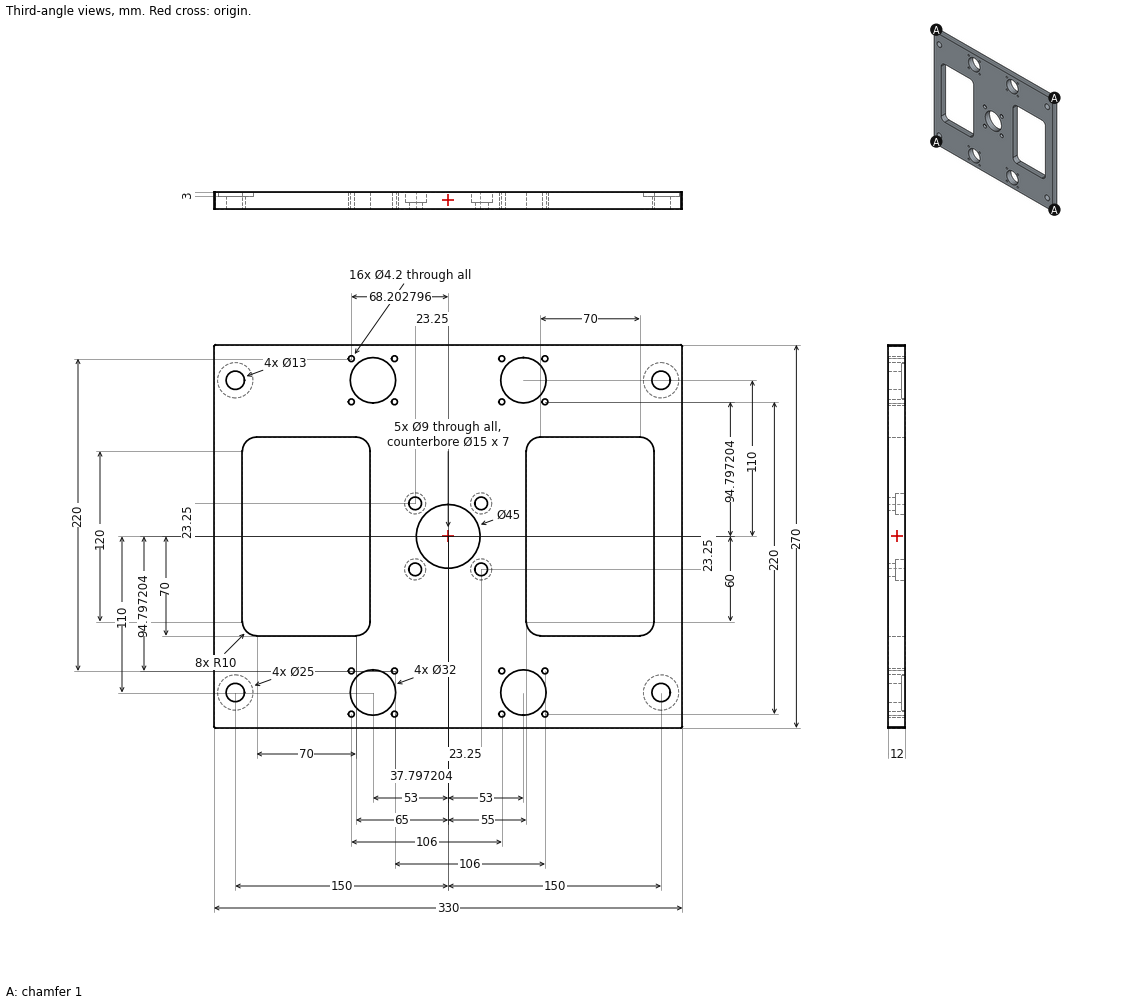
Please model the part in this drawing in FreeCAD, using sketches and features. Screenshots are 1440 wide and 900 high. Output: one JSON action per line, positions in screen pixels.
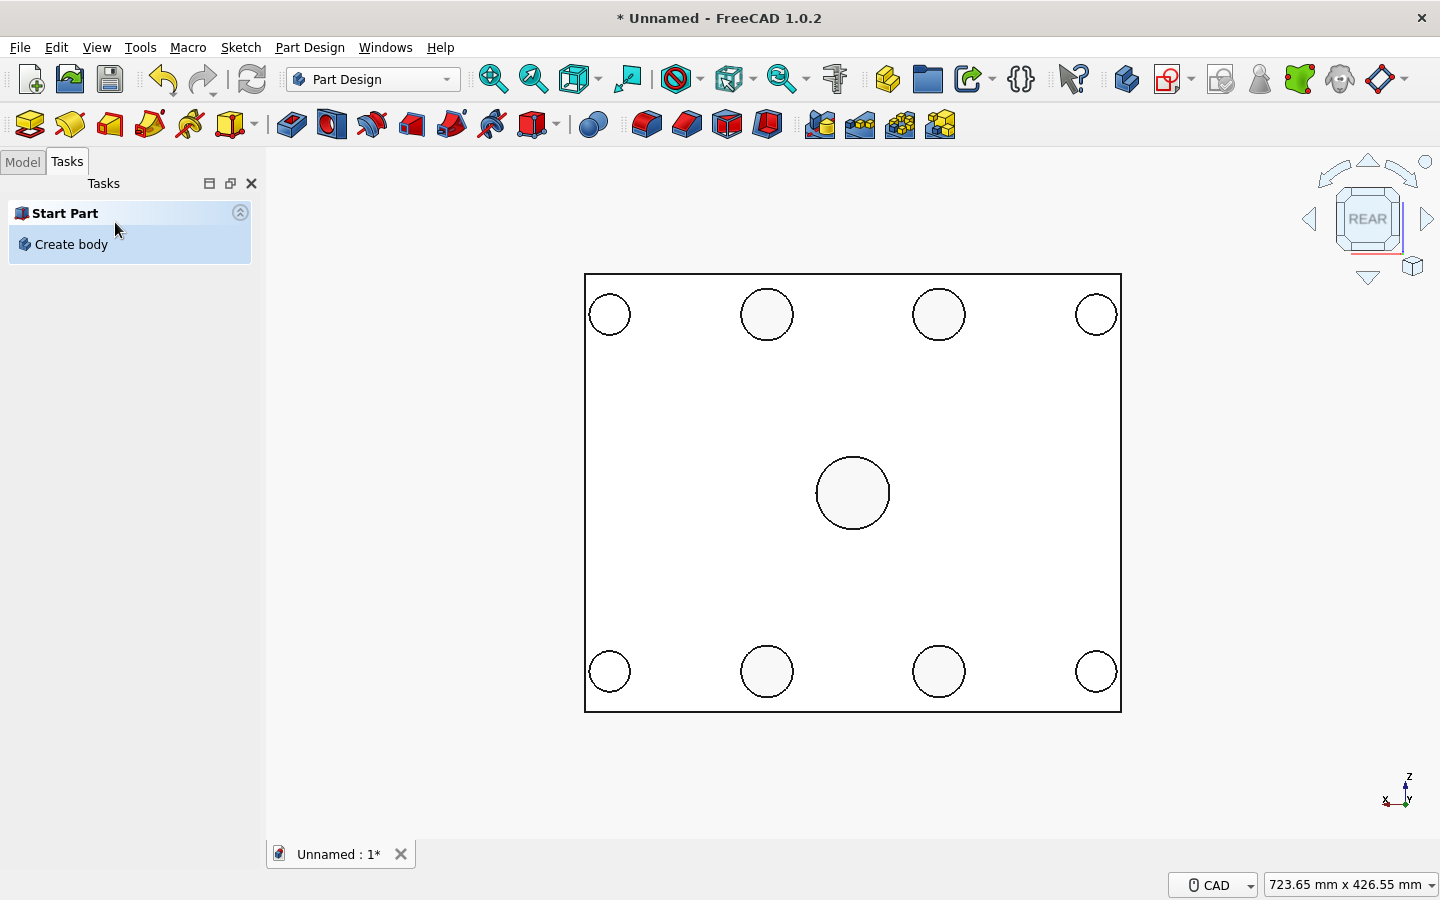
{"action": "key", "text": "0"}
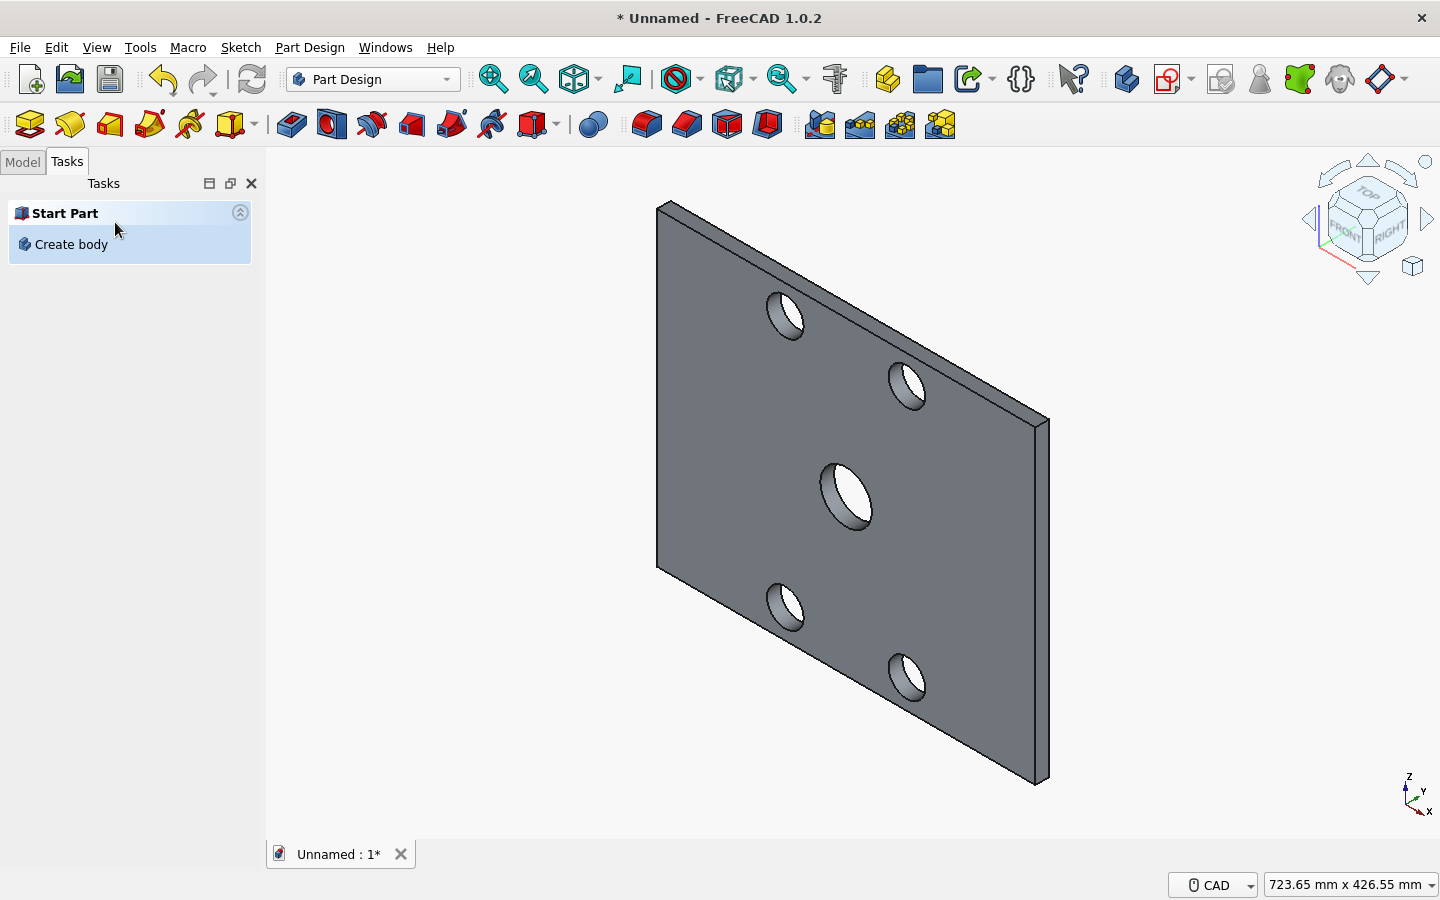
{"action": "left_click", "coordinate": [954, 558]}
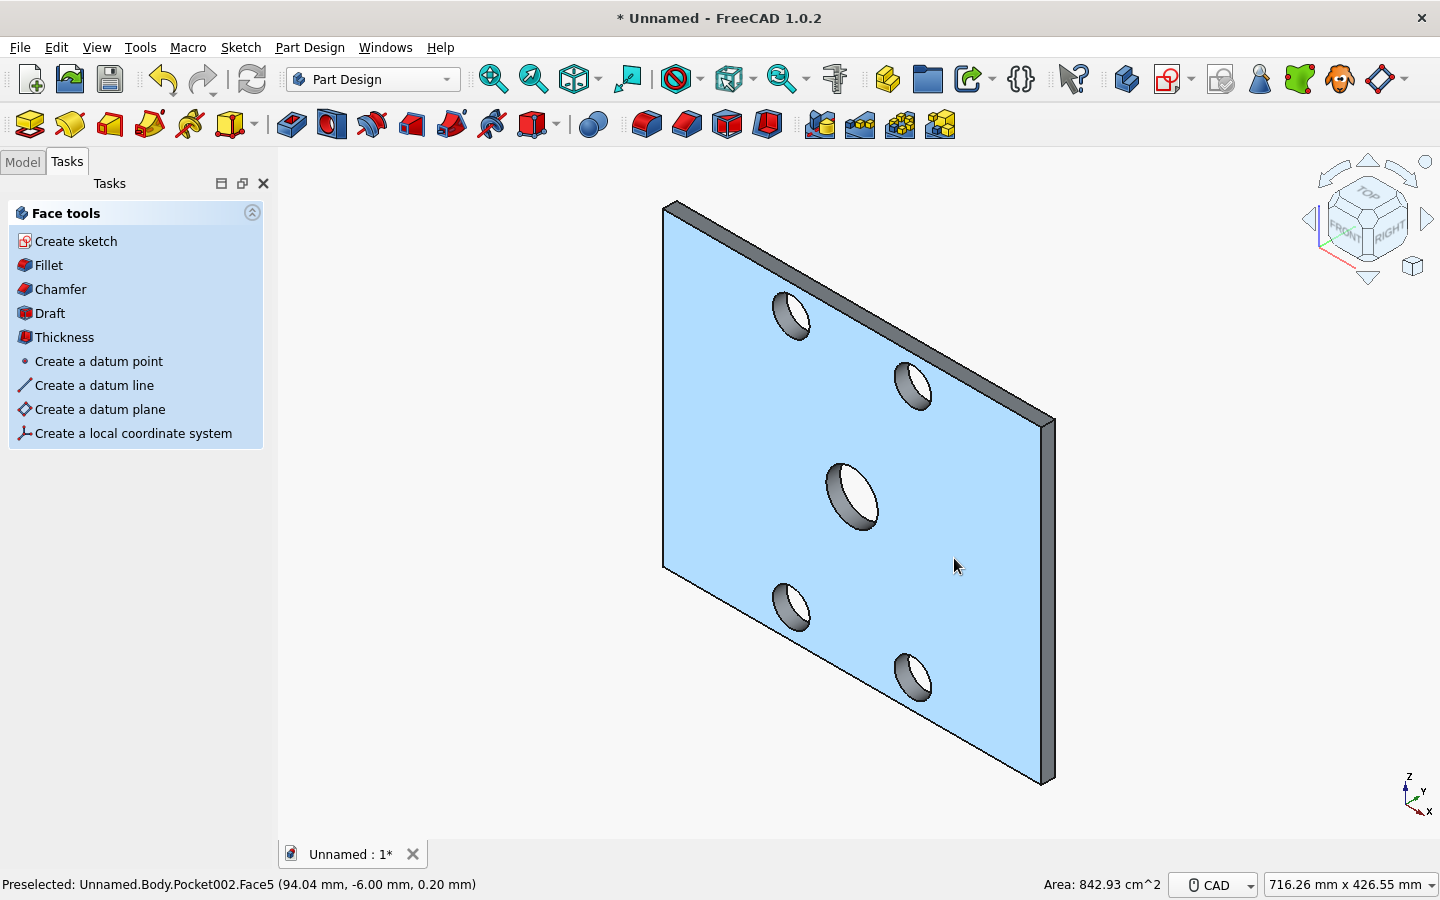
{"action": "left_click", "coordinate": [1168, 80]}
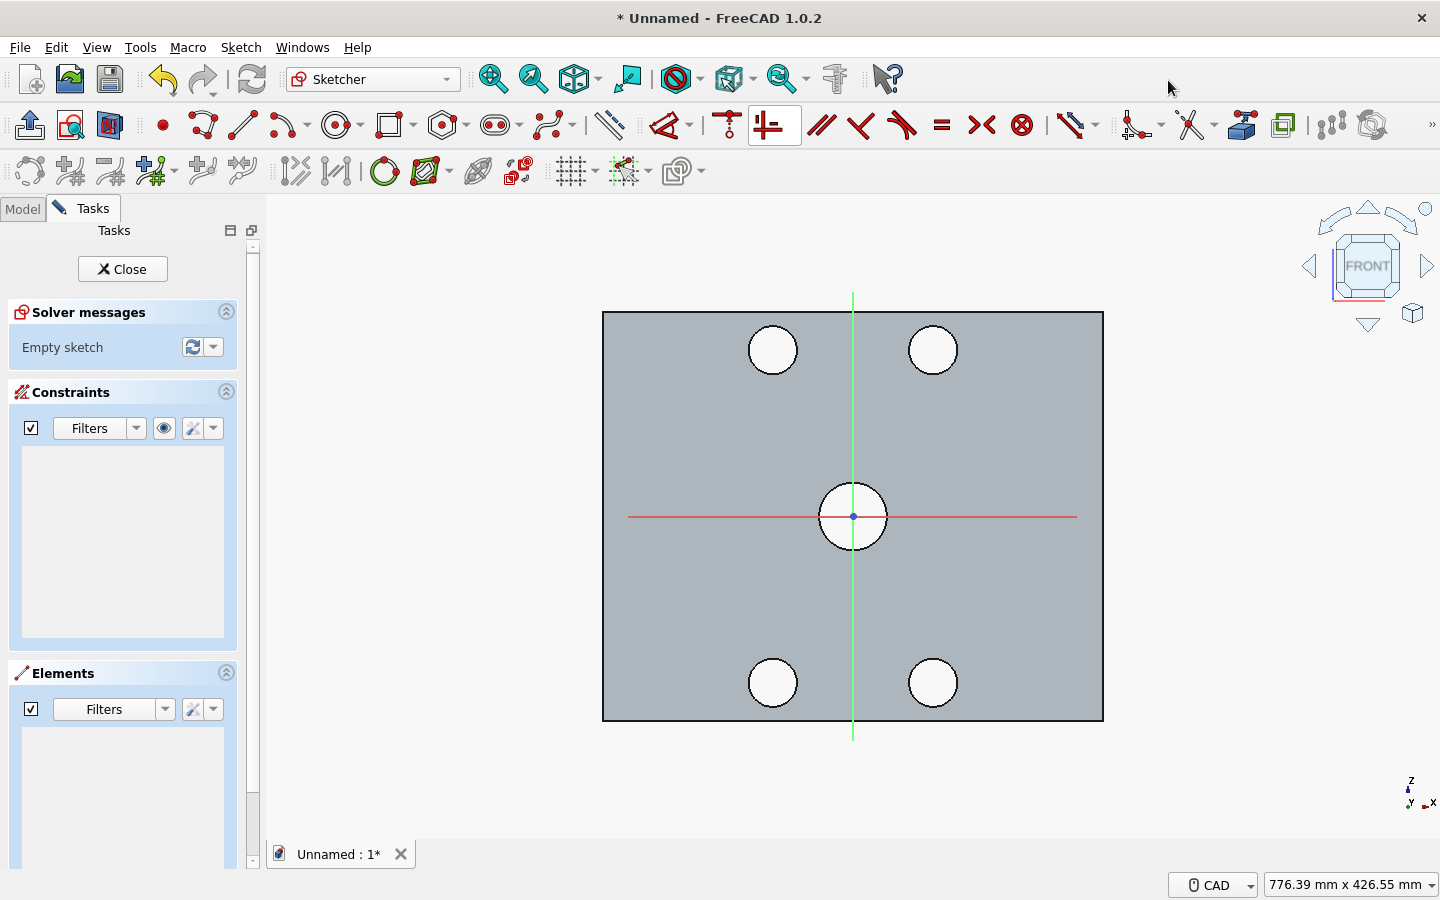
{"action": "left_click", "coordinate": [336, 126]}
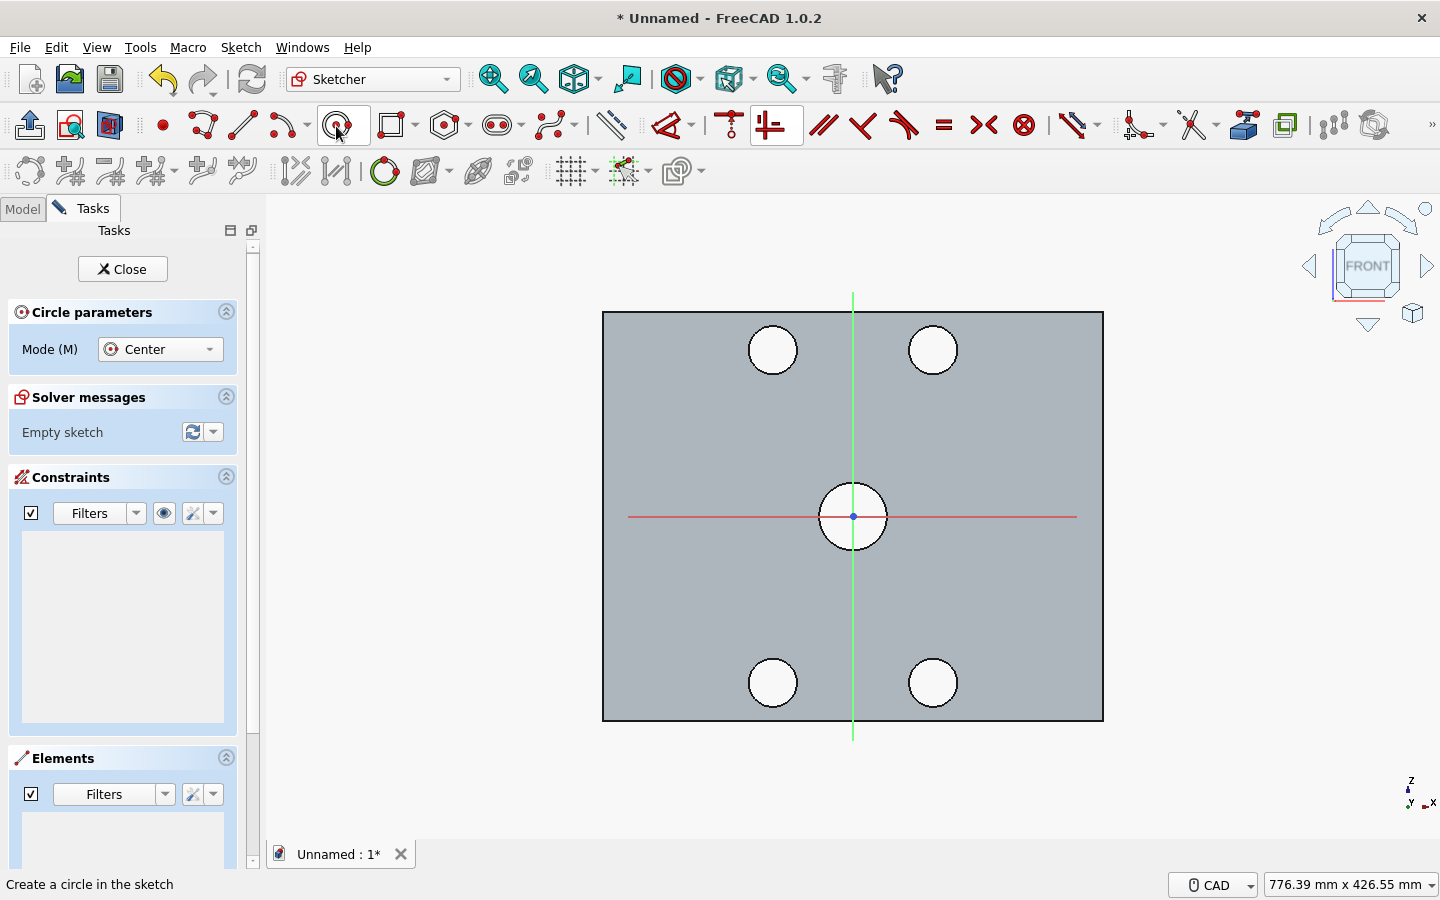
{"action": "scroll", "coordinate": [626, 350], "scroll_direction": "up", "scroll_amount": 5}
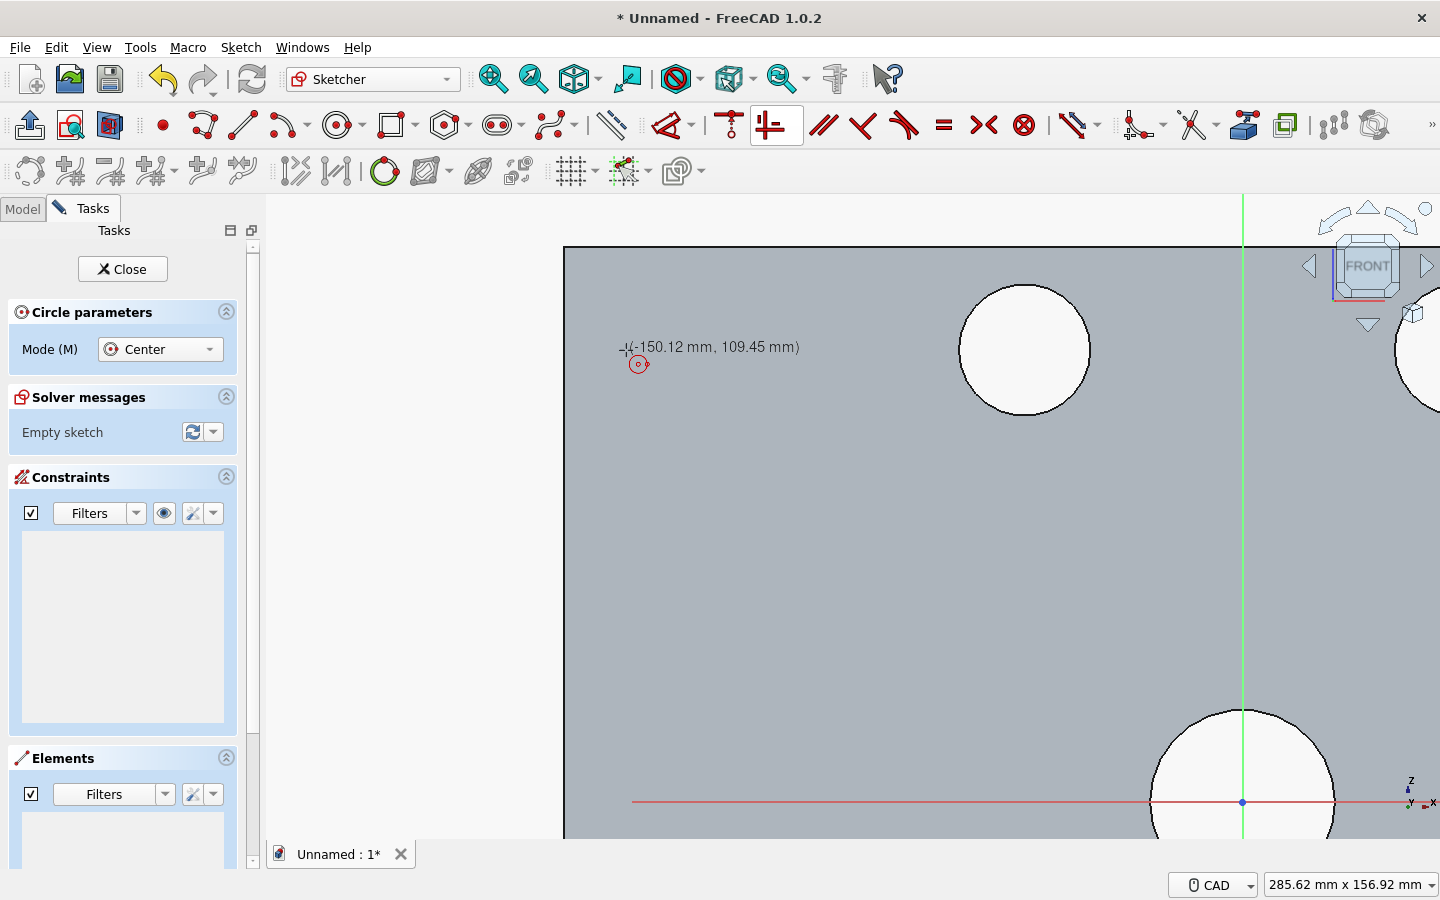
{"action": "left_click", "coordinate": [626, 350]}
{"action": "mouse_move", "coordinate": [645, 331]}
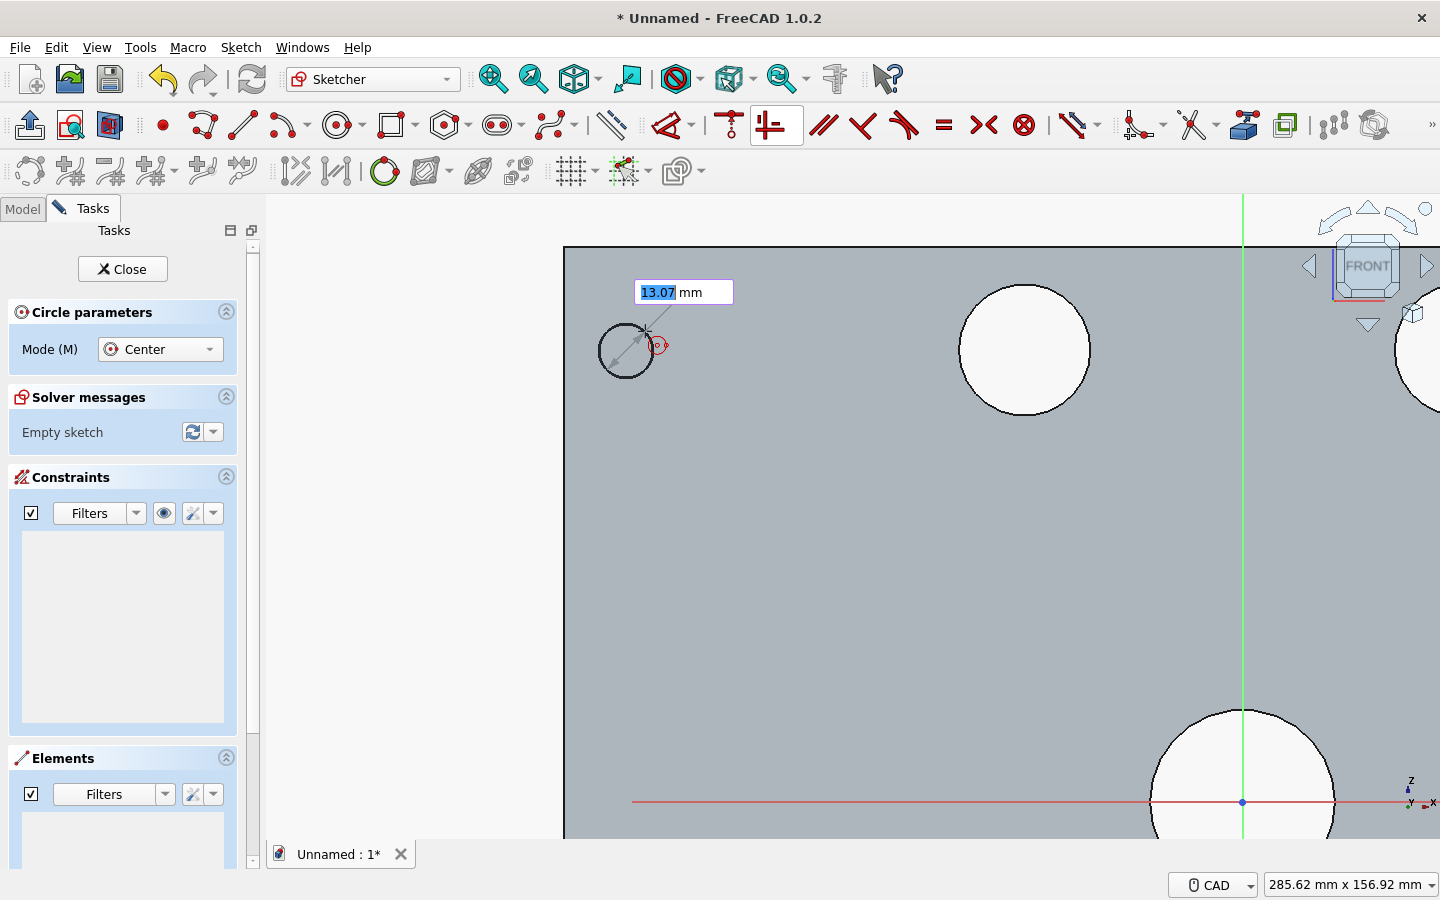
{"action": "type", "text": "13"}
{"action": "key", "text": "Return"}